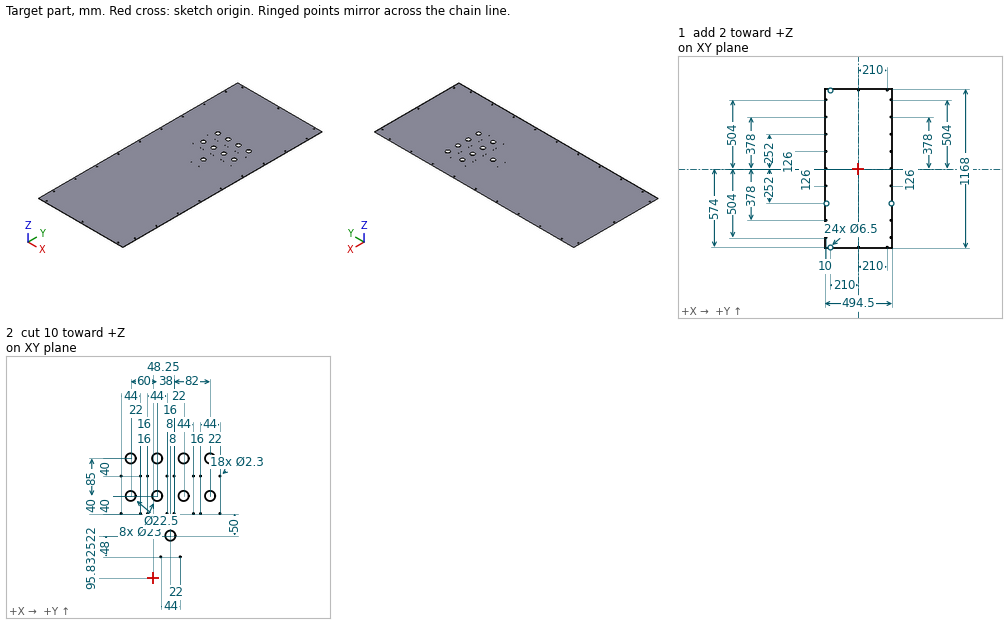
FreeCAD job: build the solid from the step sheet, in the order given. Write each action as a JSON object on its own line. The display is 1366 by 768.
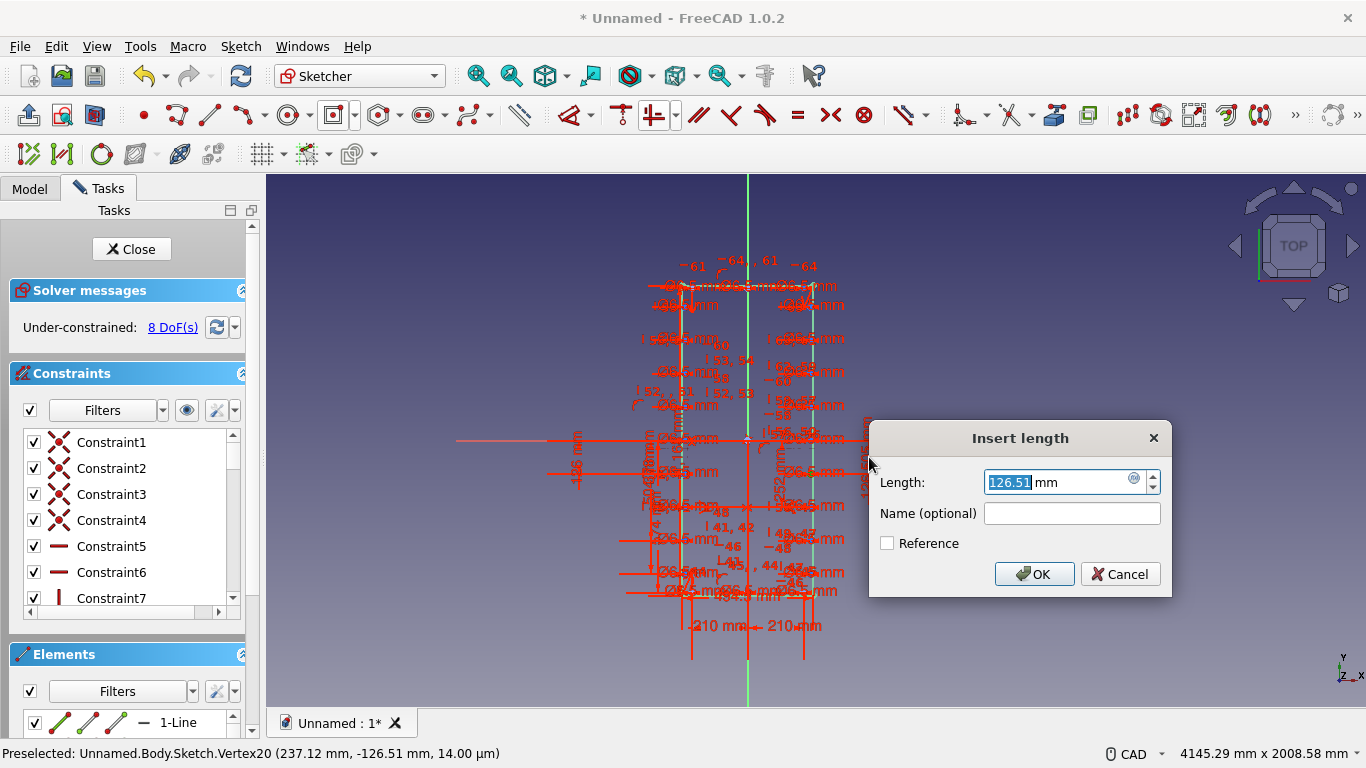
{"action": "type", "text": "126"}
{"action": "key", "text": "Return"}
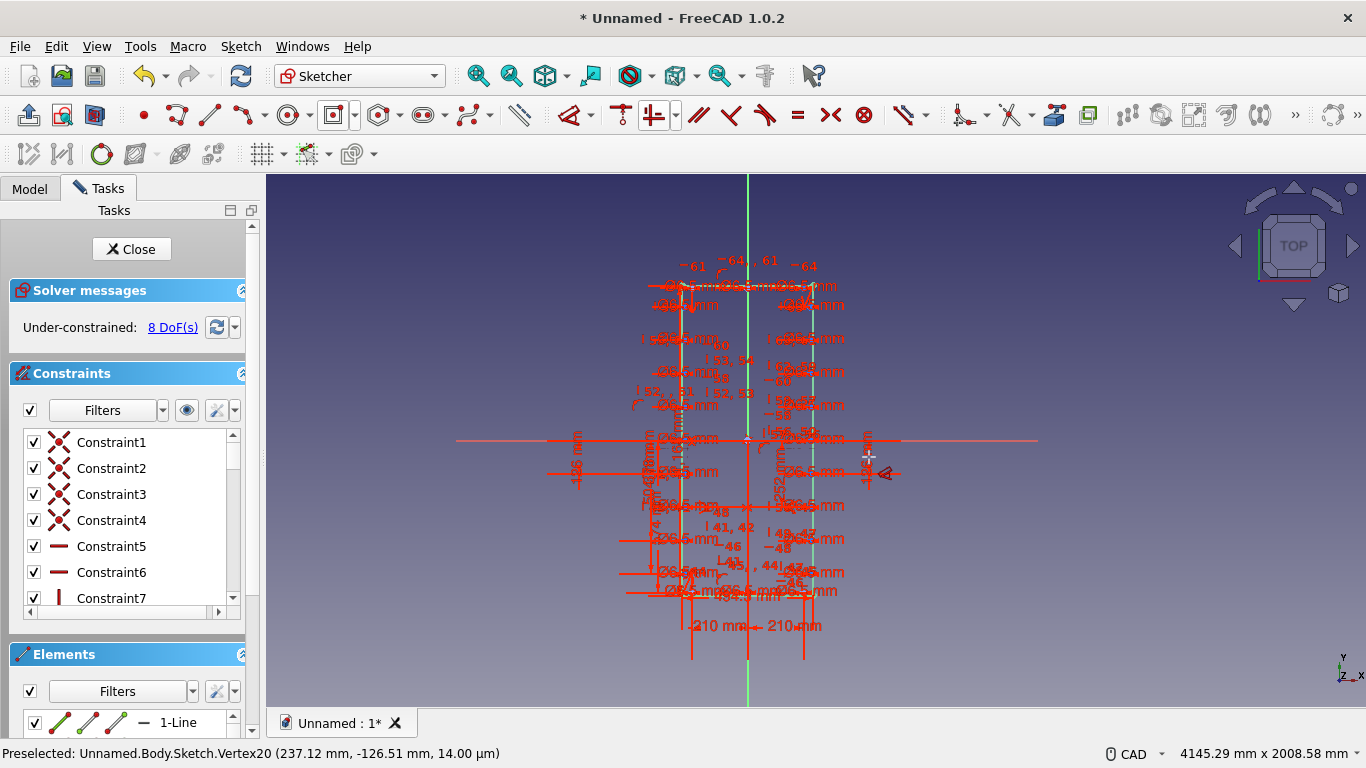
{"action": "left_click", "coordinate": [685, 407]}
{"action": "left_click", "coordinate": [651, 424]}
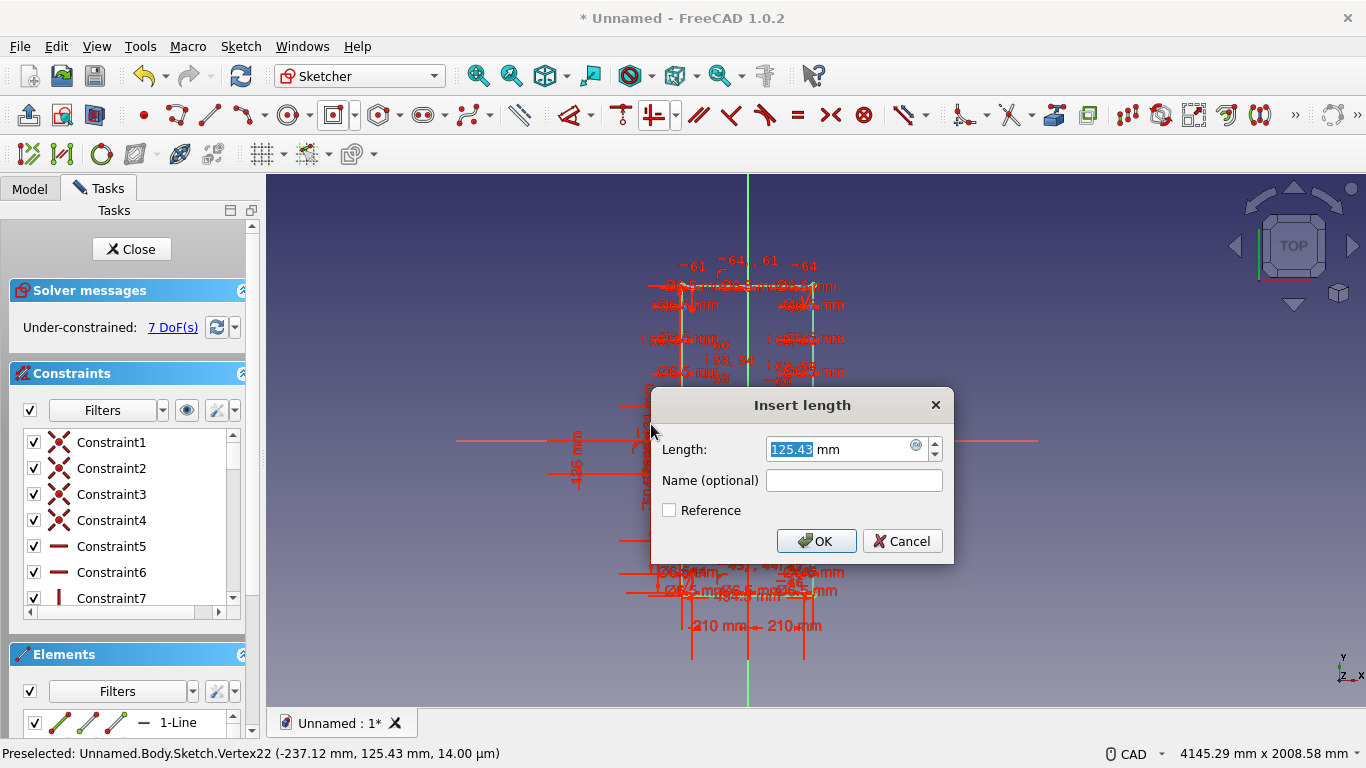
{"action": "type", "text": "126"}
{"action": "key", "text": "Return"}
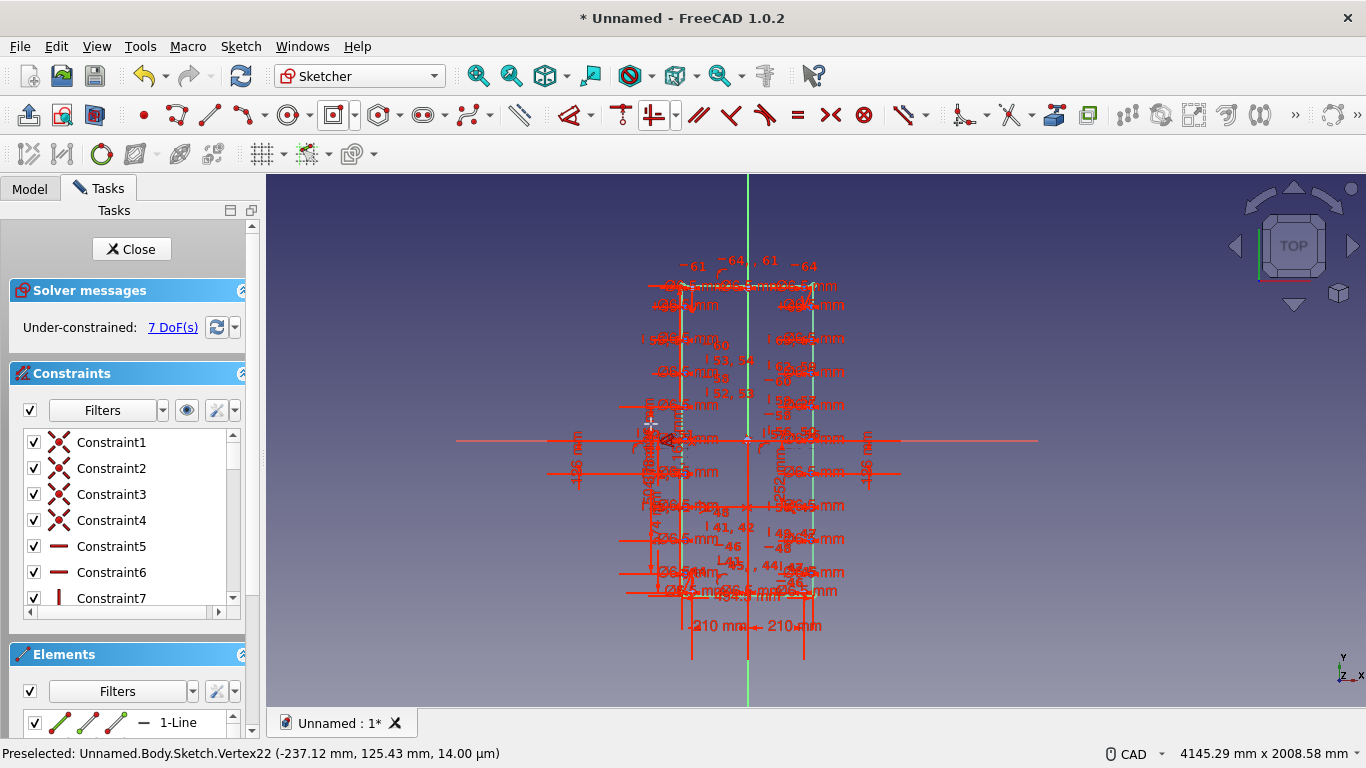
{"action": "left_click", "coordinate": [685, 374]}
{"action": "left_click", "coordinate": [651, 392]}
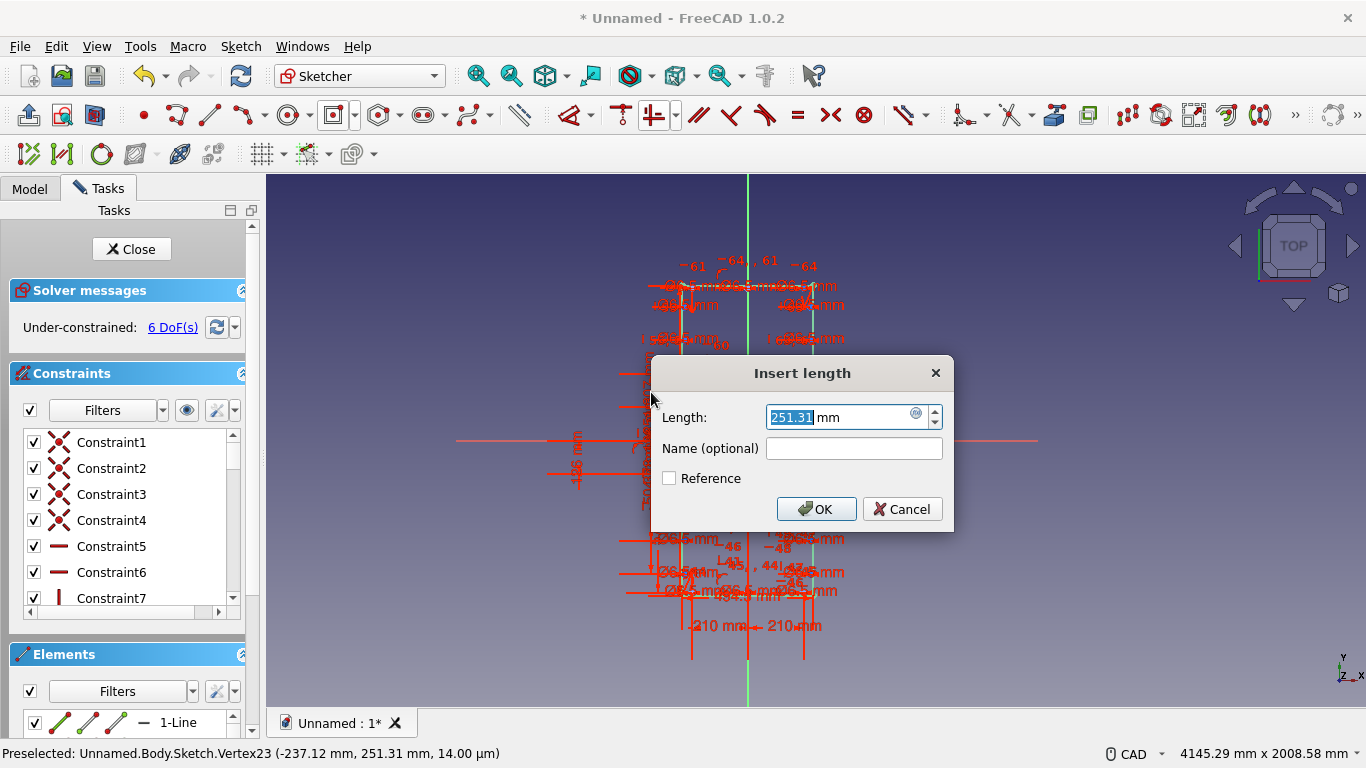
{"action": "type", "text": "252"}
{"action": "key", "text": "Return"}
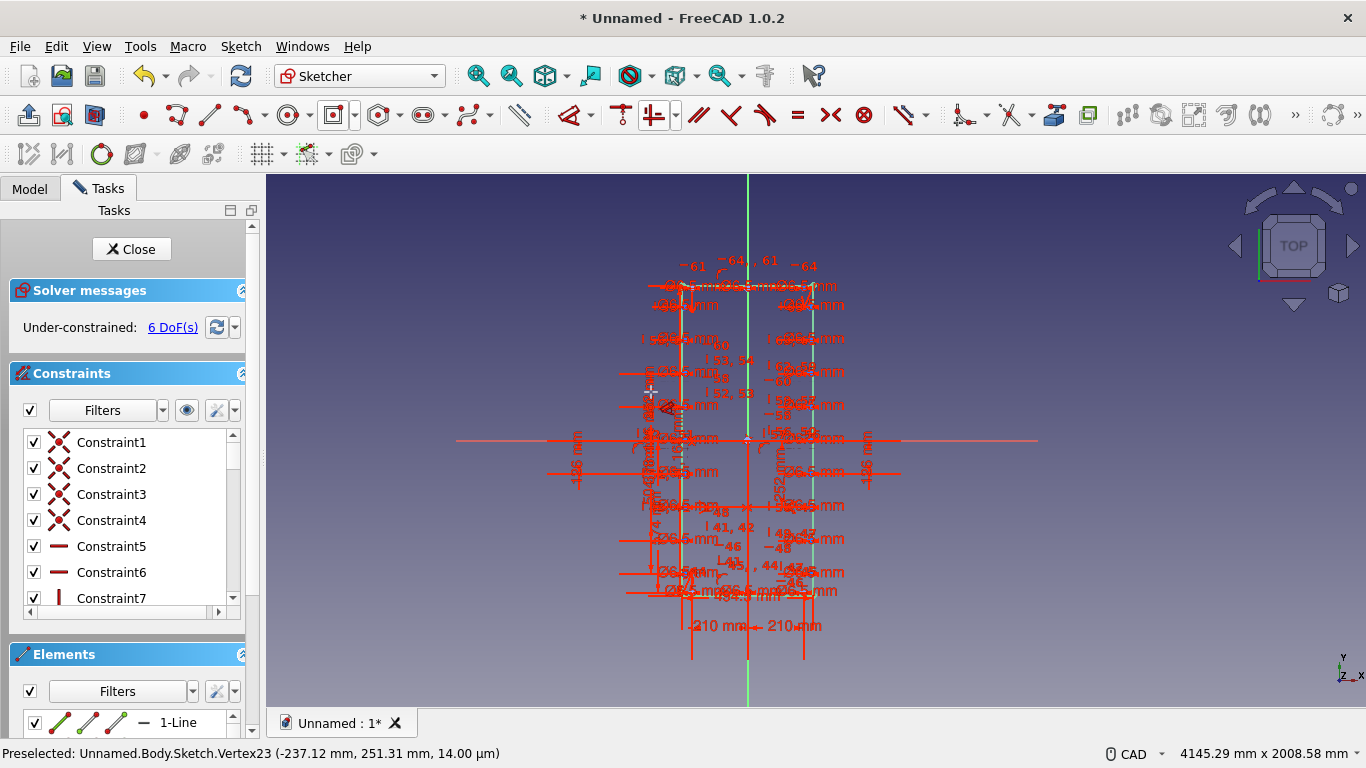
{"action": "left_click", "coordinate": [685, 340]}
{"action": "left_click", "coordinate": [651, 367]}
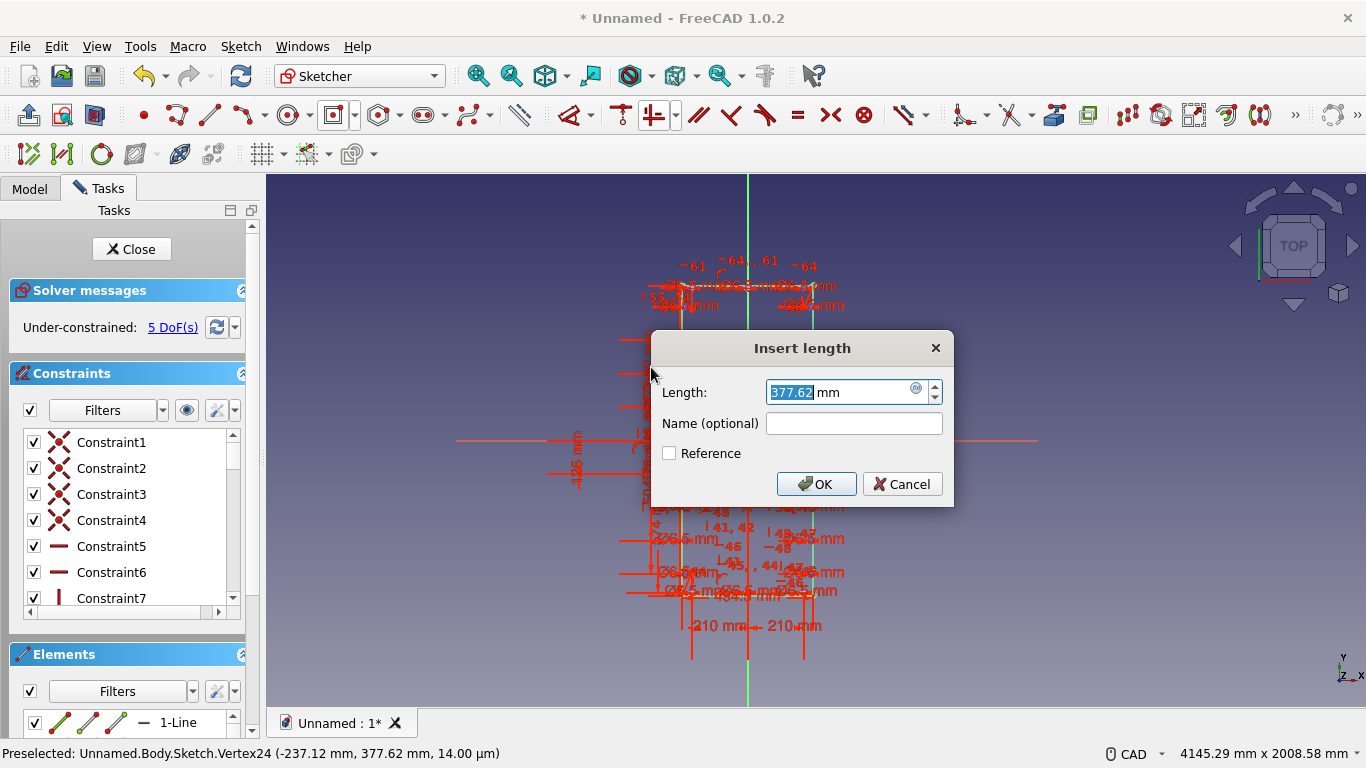
{"action": "type", "text": "378"}
{"action": "key", "text": "Return"}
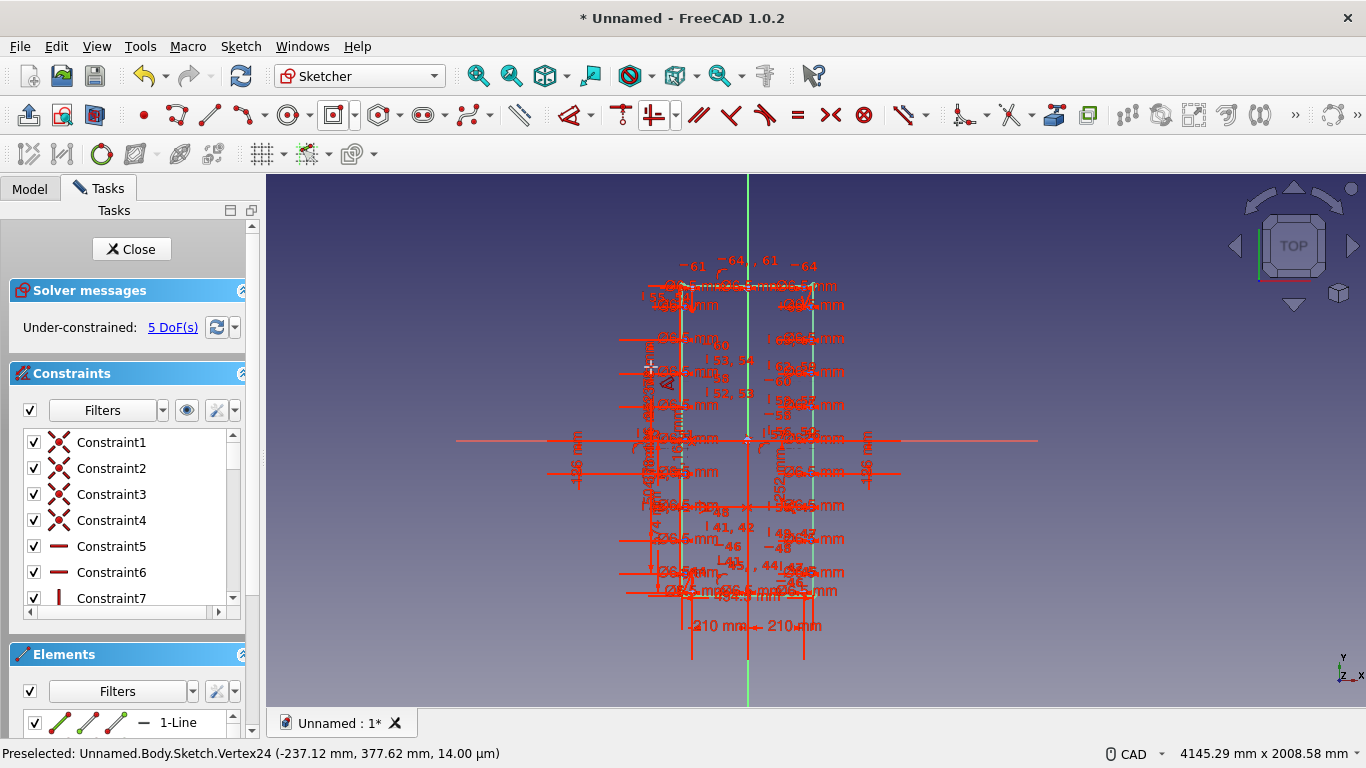
{"action": "left_click", "coordinate": [685, 307]}
{"action": "left_click", "coordinate": [651, 343]}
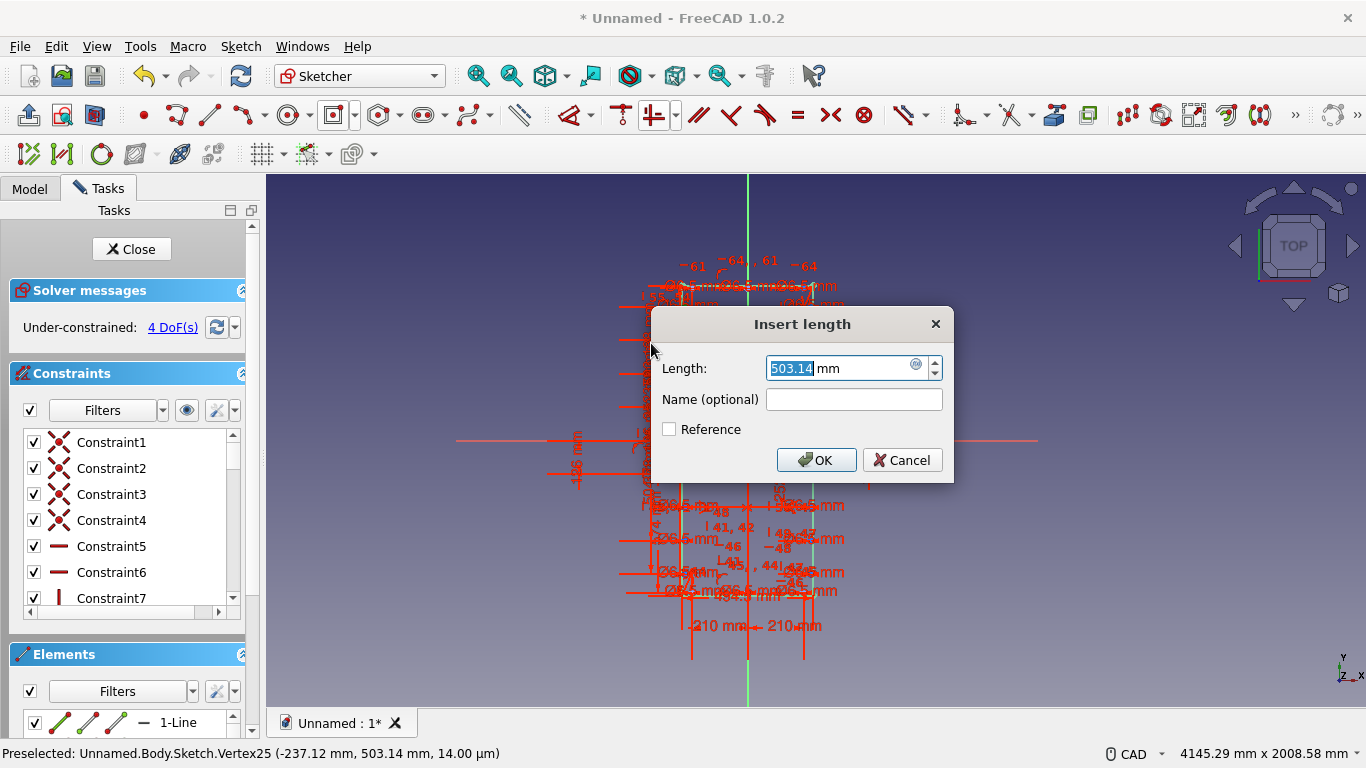
{"action": "type", "text": "504"}
{"action": "key", "text": "Return"}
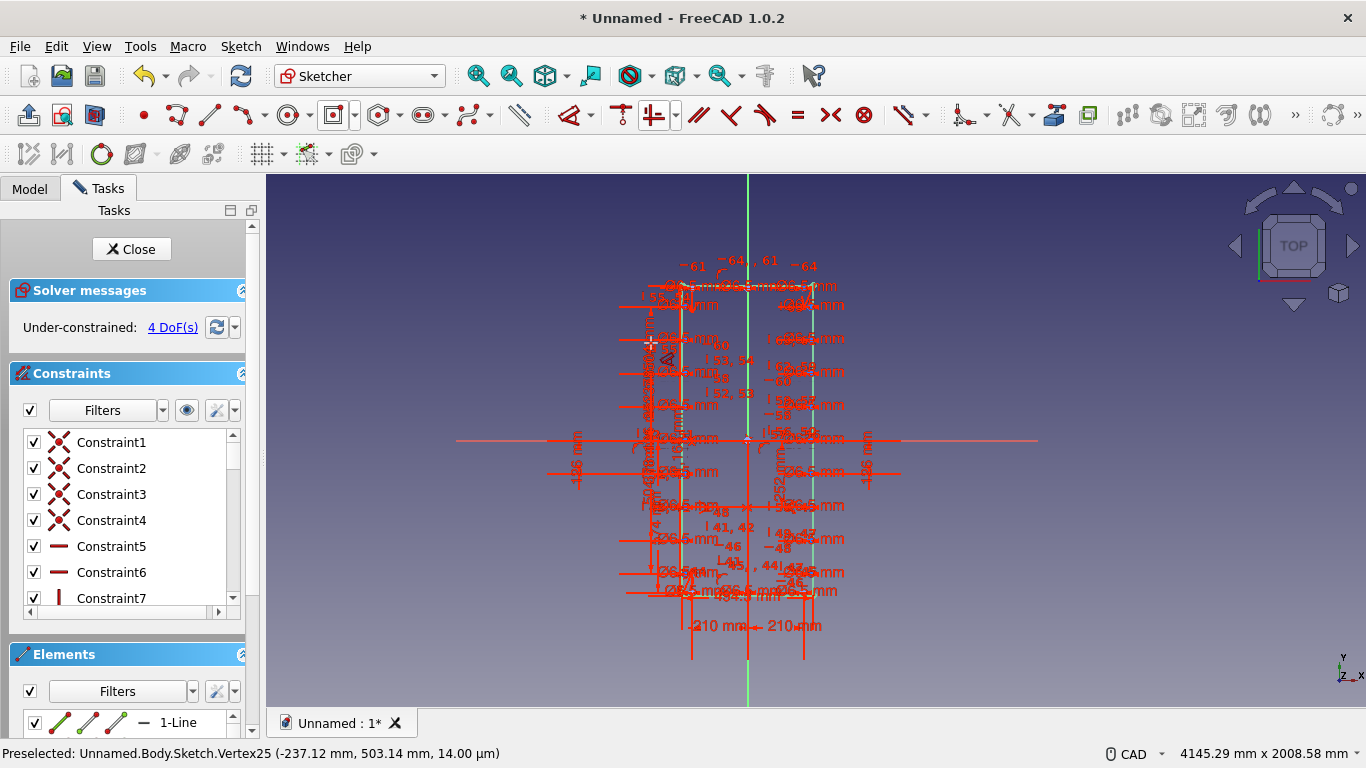
{"action": "left_click", "coordinate": [811, 340]}
{"action": "left_click", "coordinate": [845, 391]}